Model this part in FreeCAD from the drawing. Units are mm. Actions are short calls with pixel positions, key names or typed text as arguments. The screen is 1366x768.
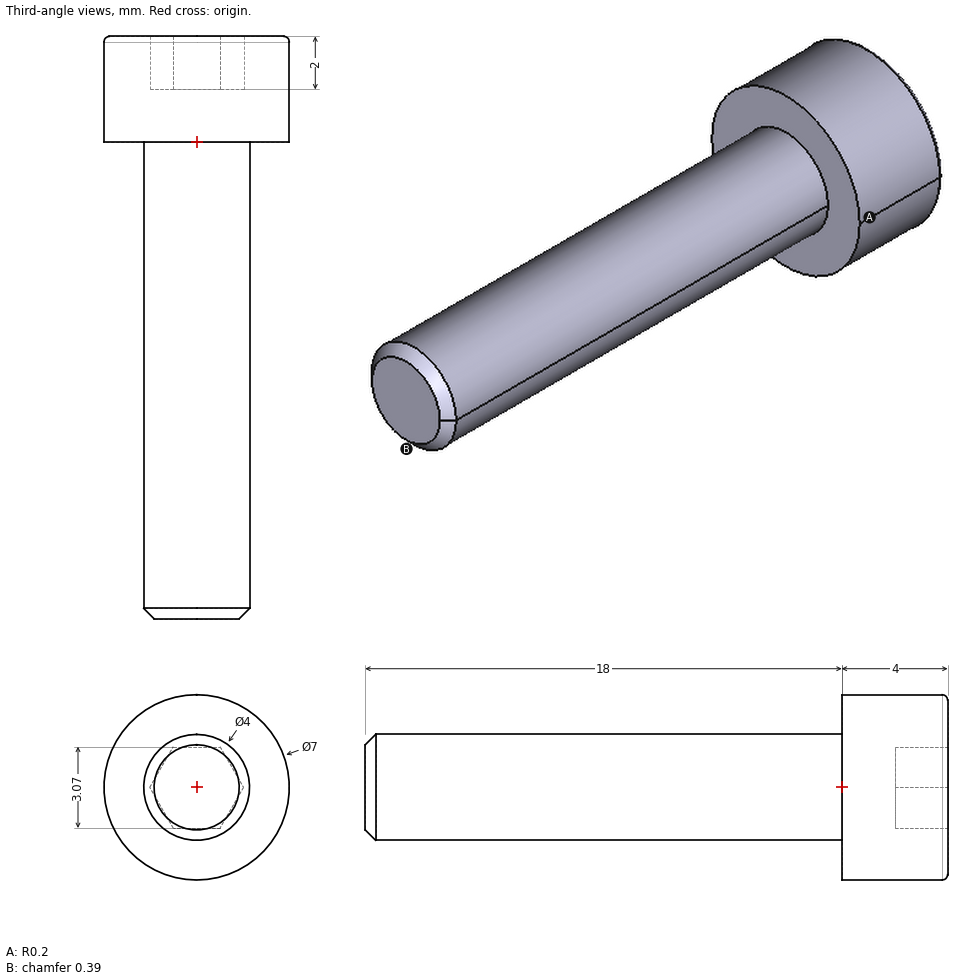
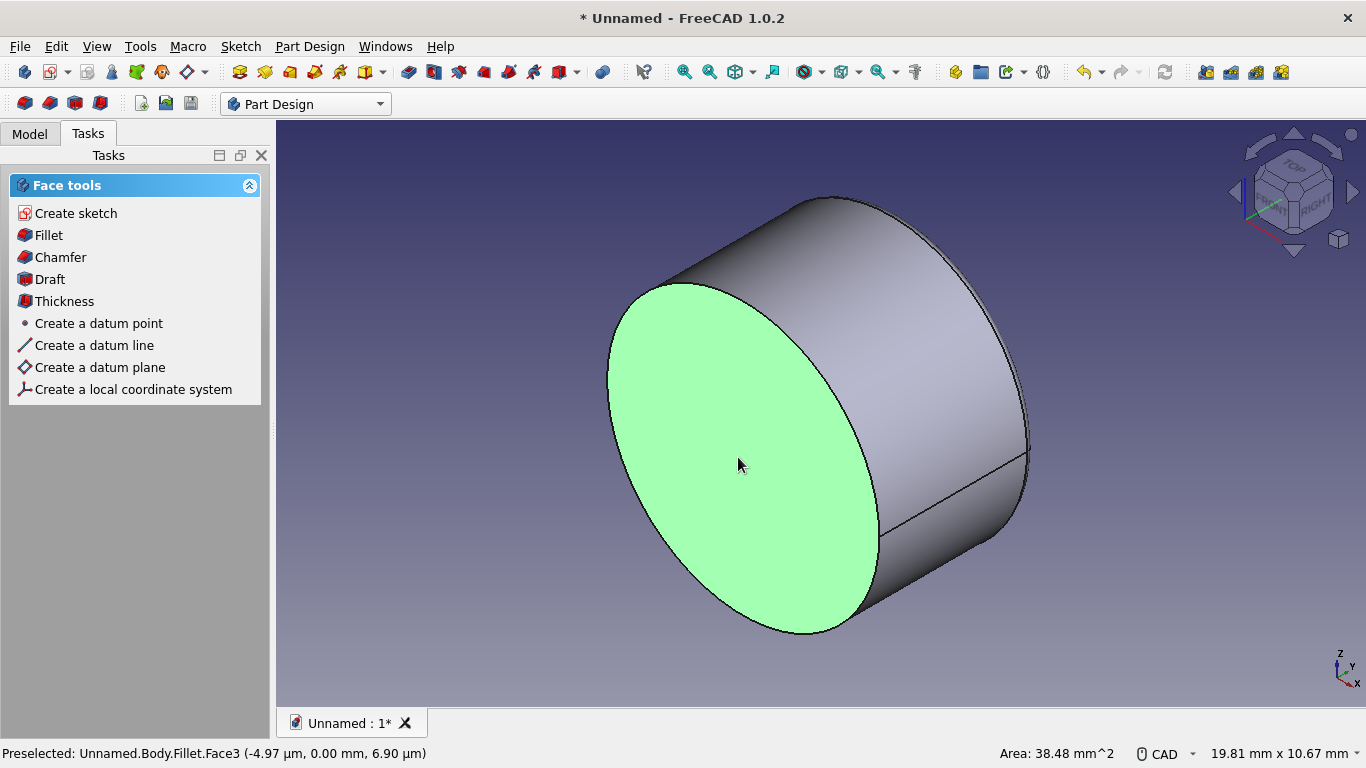
click(50, 72)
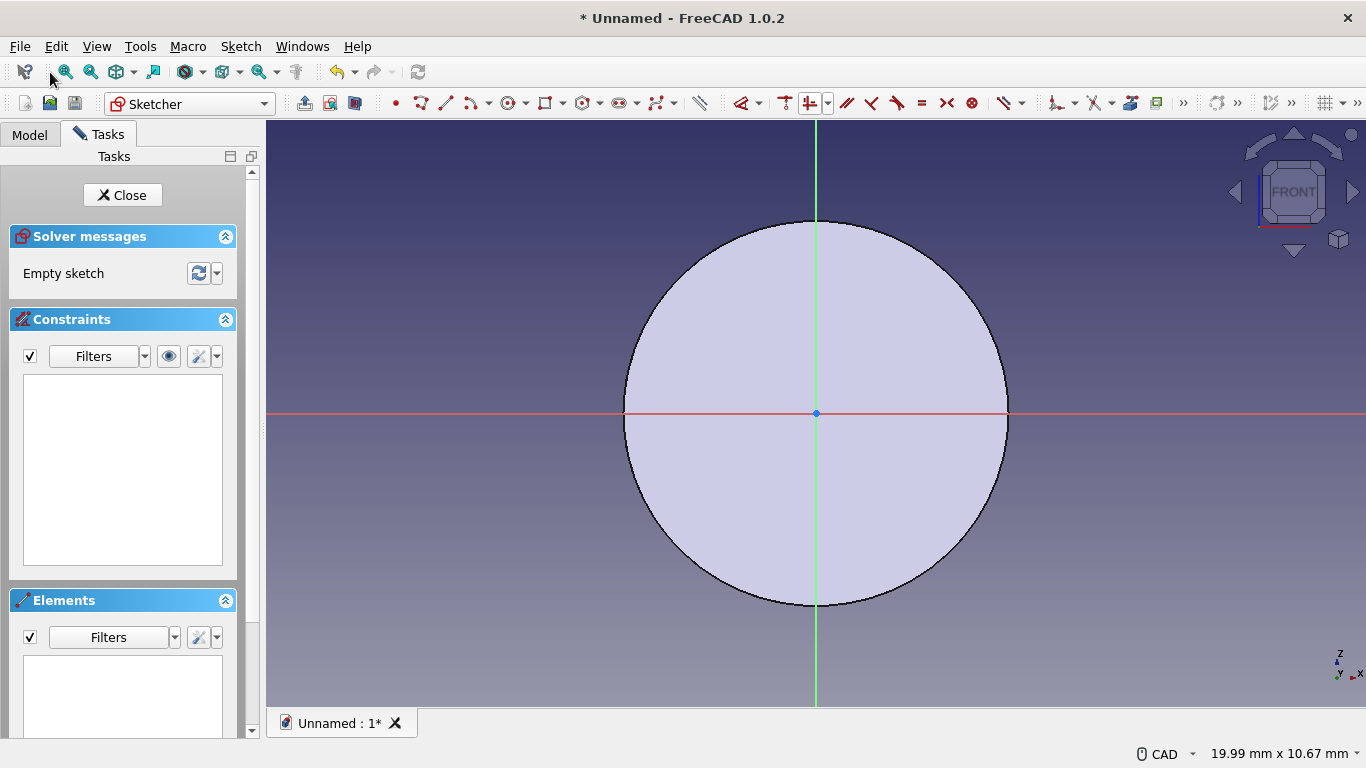
scroll(899, 414, up, 3)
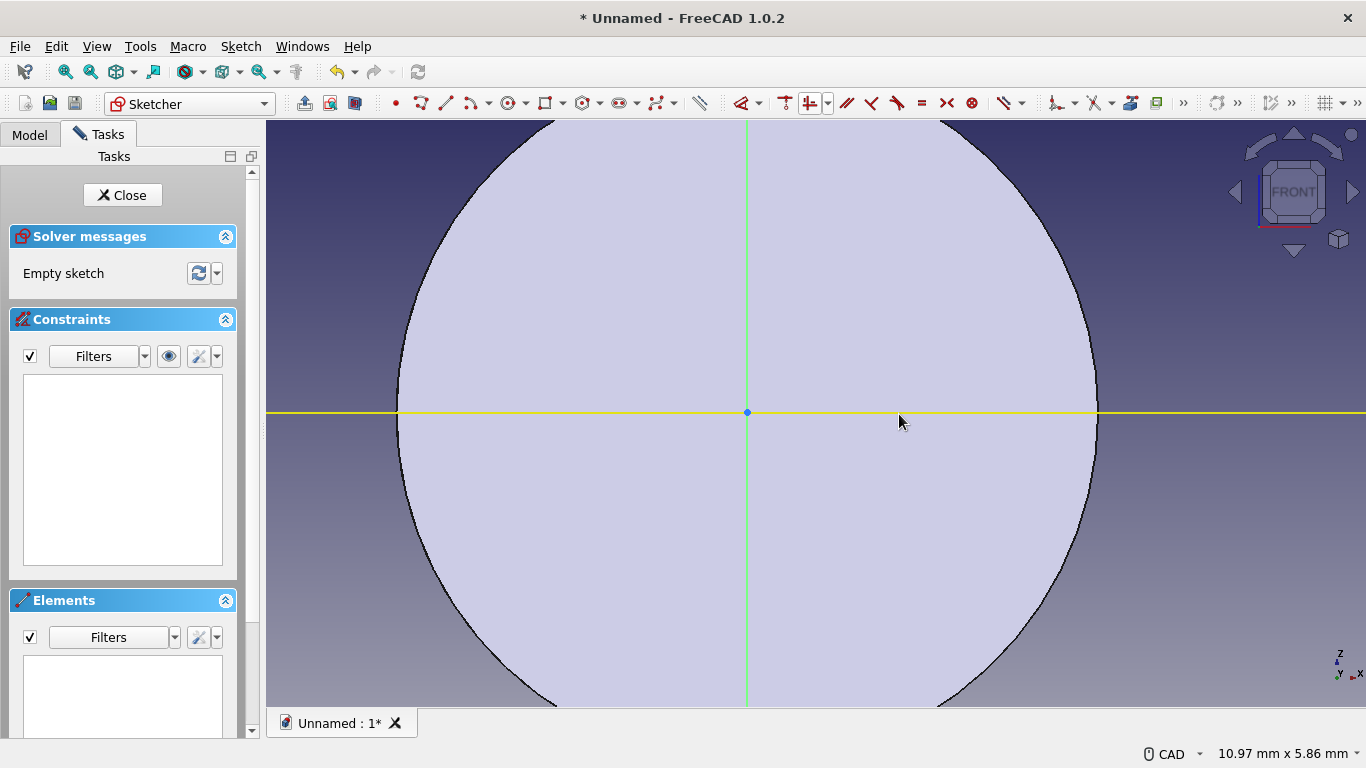
click(508, 104)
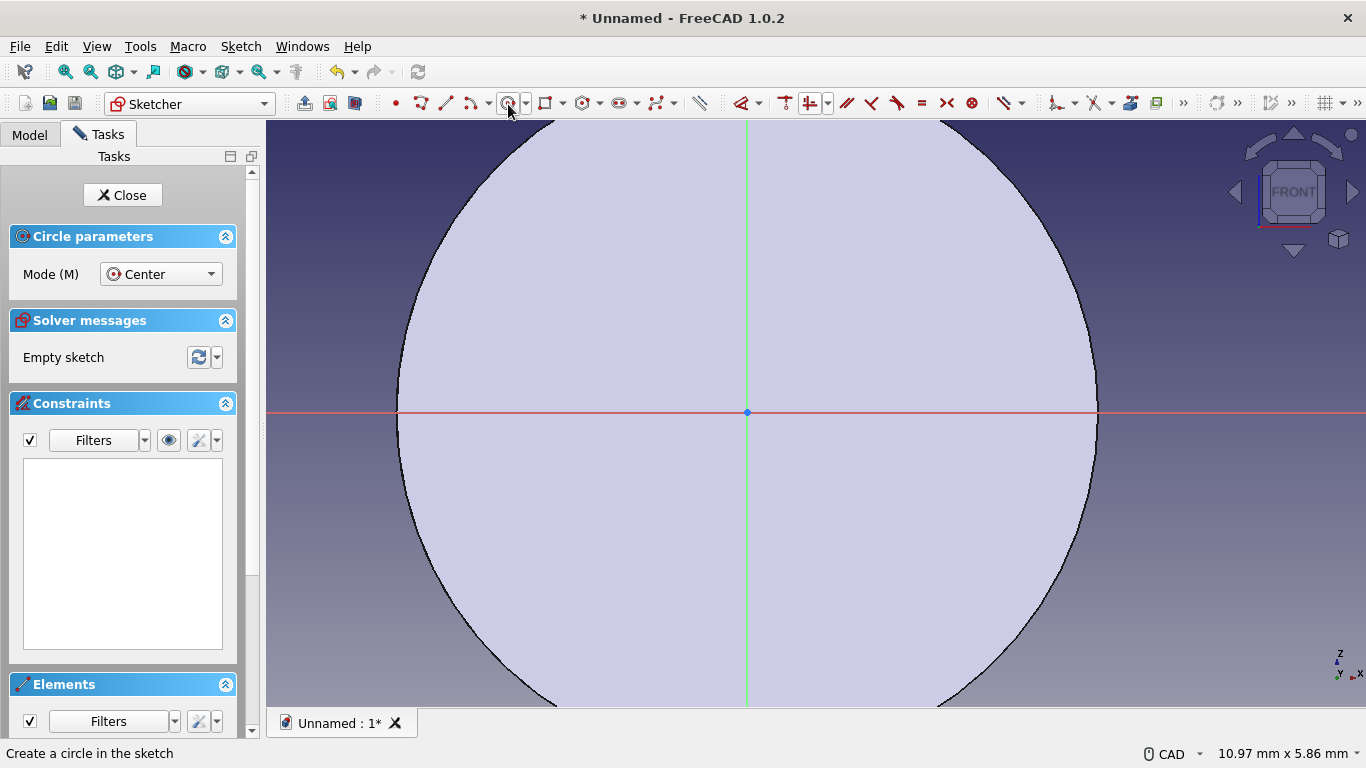
click(747, 413)
click(889, 271)
key(Escape)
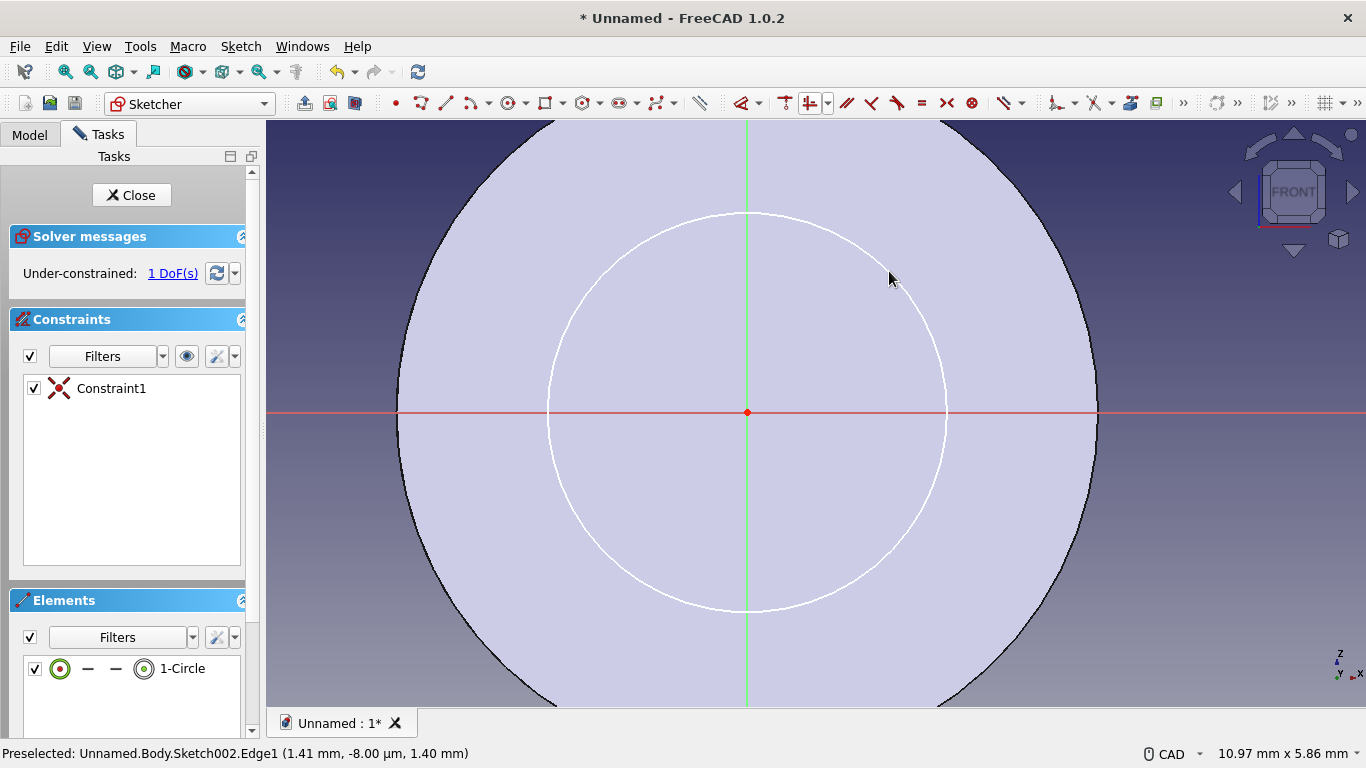
click(740, 104)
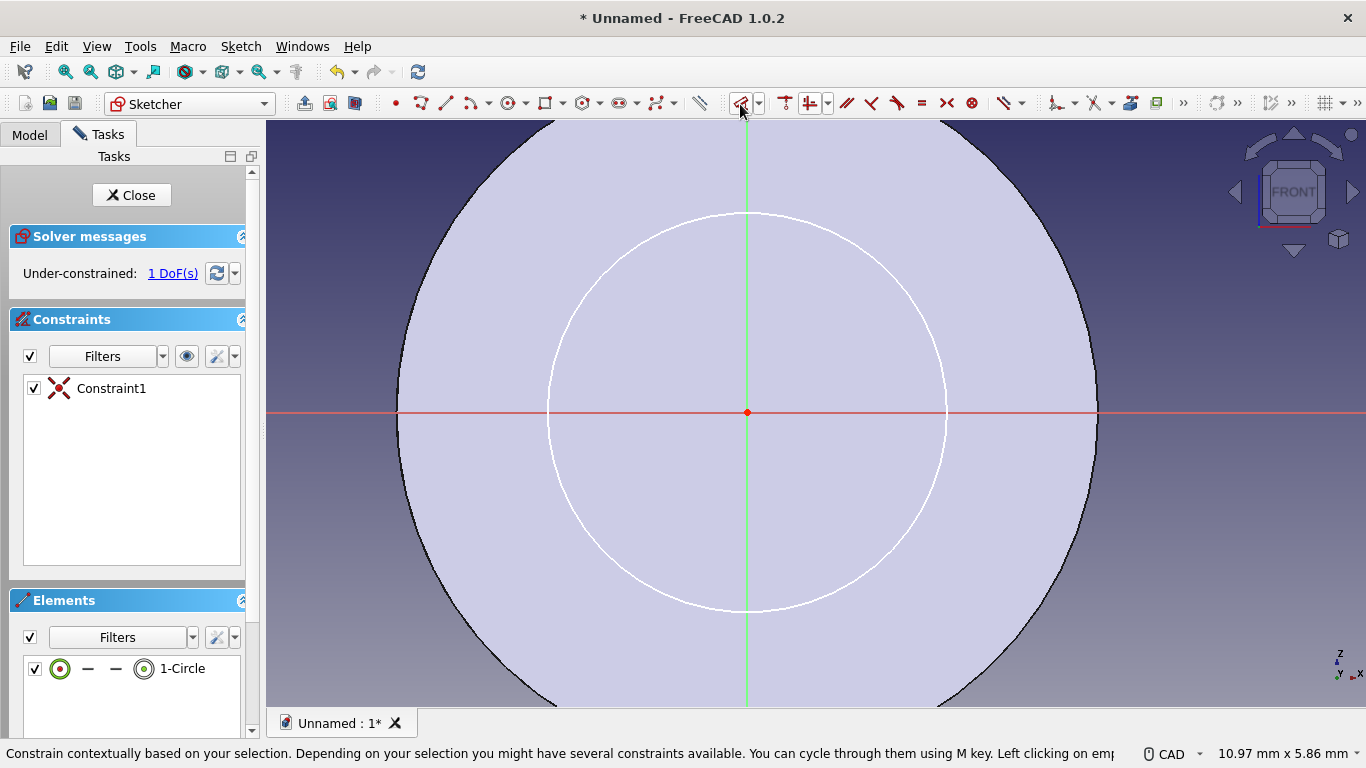
click(888, 271)
click(911, 248)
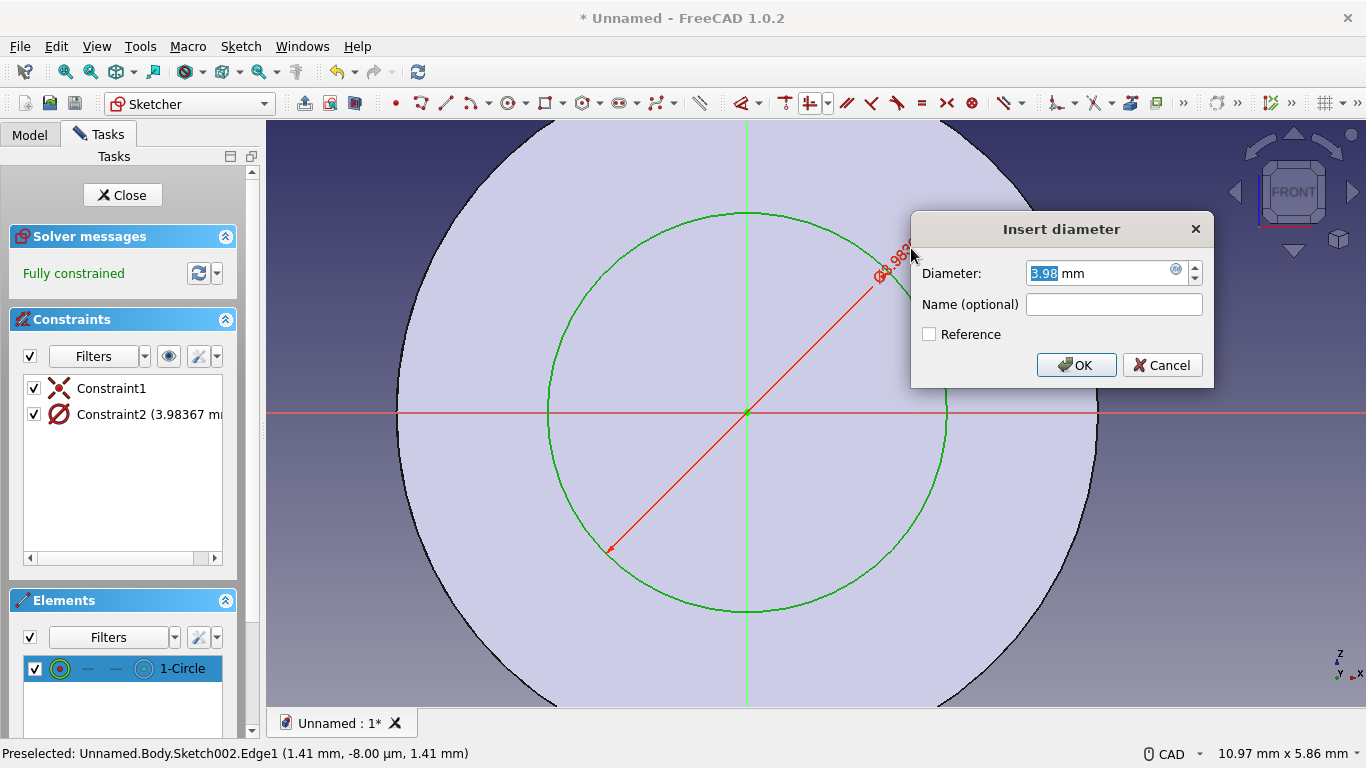
text(4)
key(Return)
key(Escape)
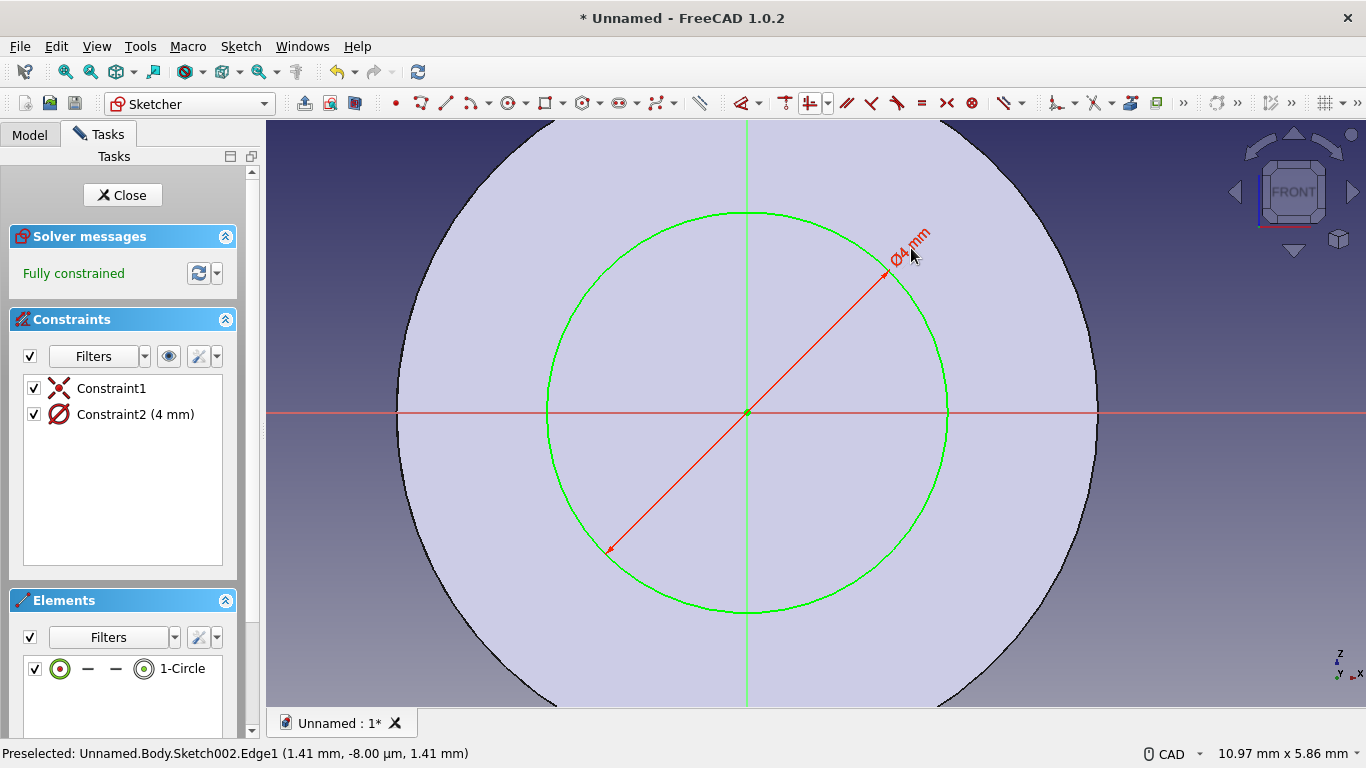
click(123, 195)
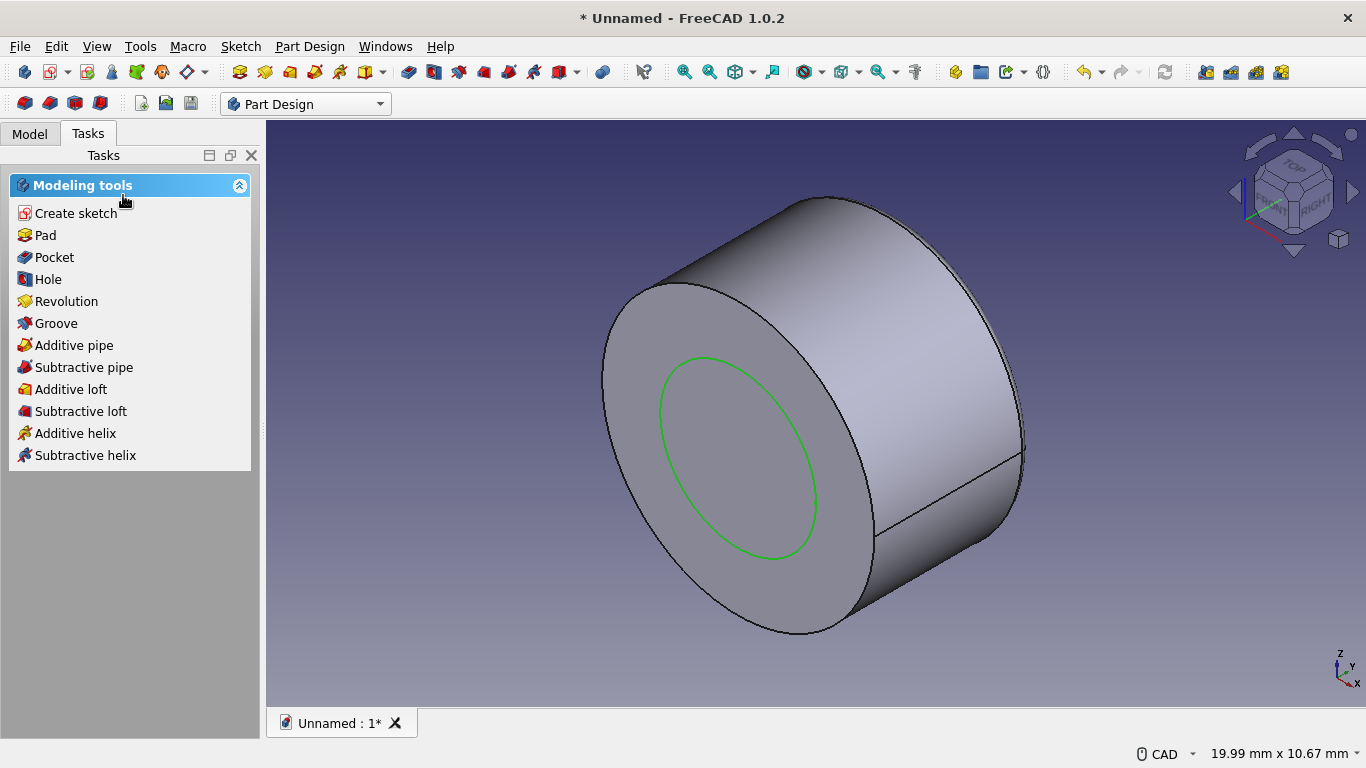
click(240, 72)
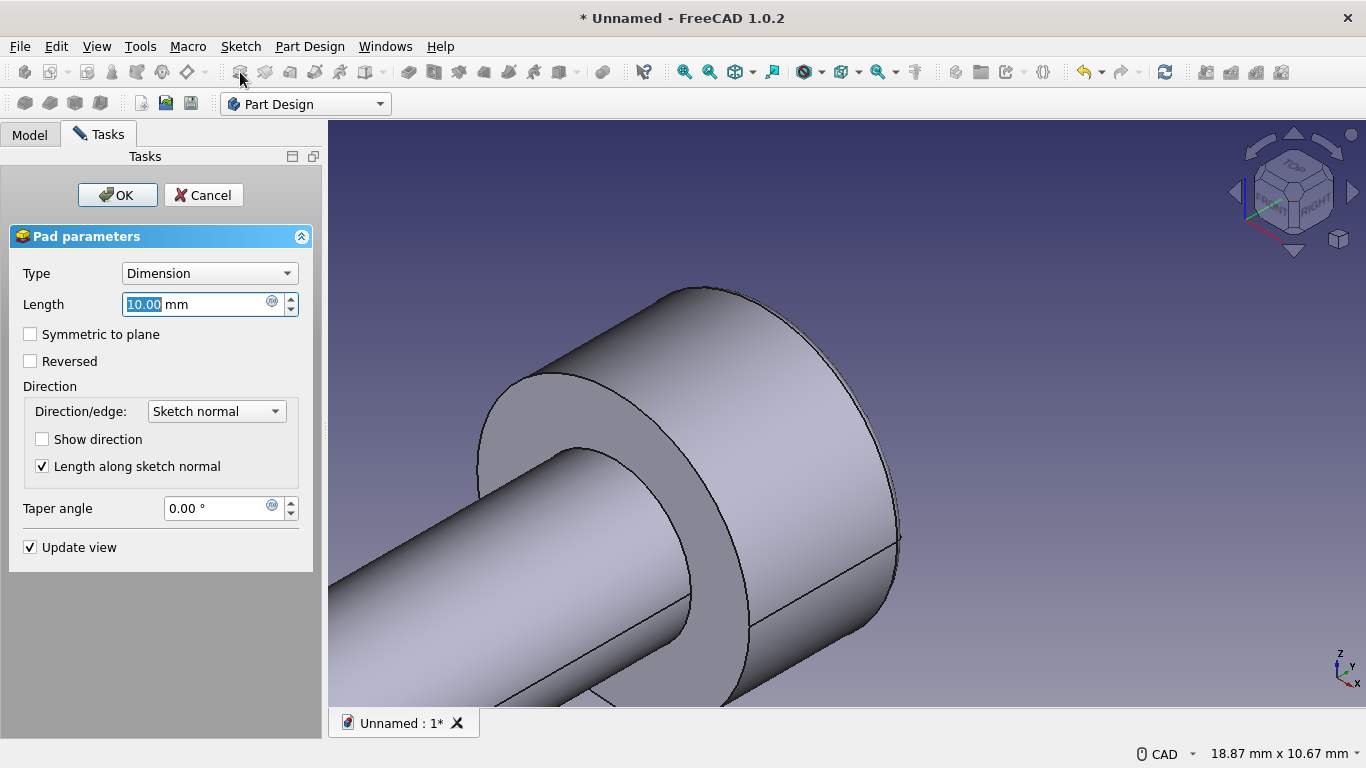
text(18)
key(Tab)